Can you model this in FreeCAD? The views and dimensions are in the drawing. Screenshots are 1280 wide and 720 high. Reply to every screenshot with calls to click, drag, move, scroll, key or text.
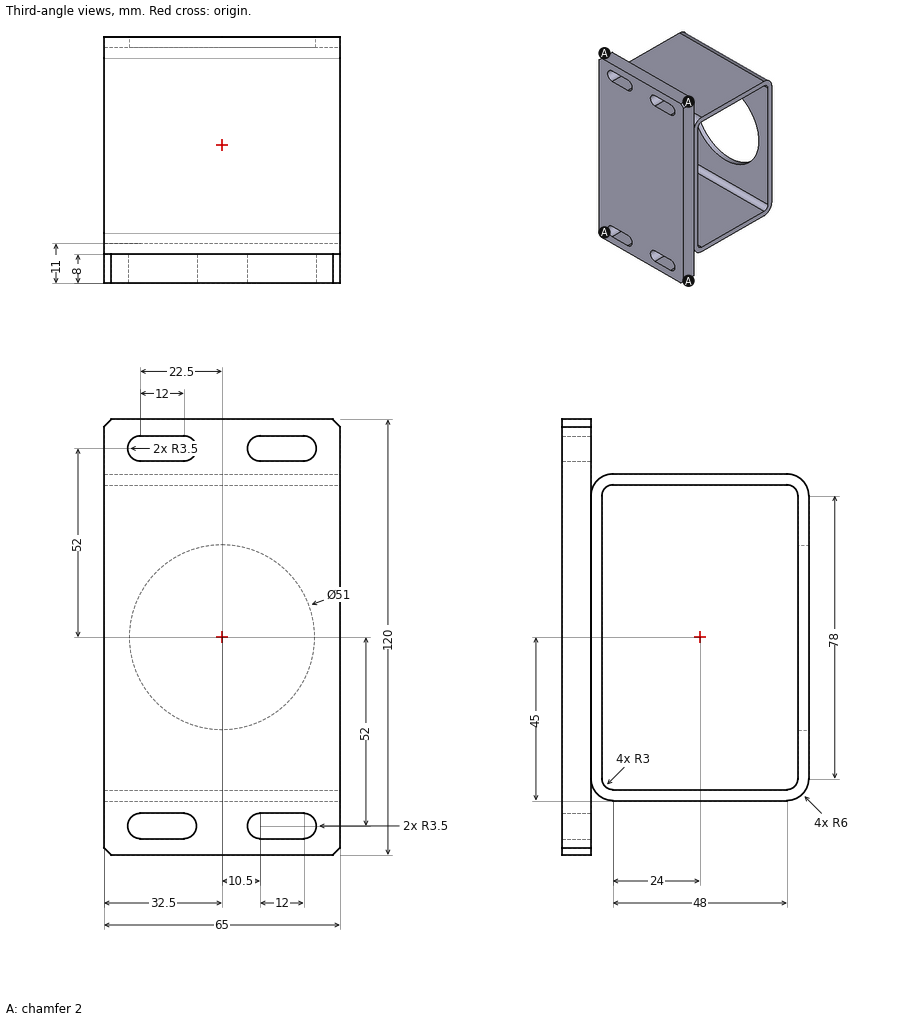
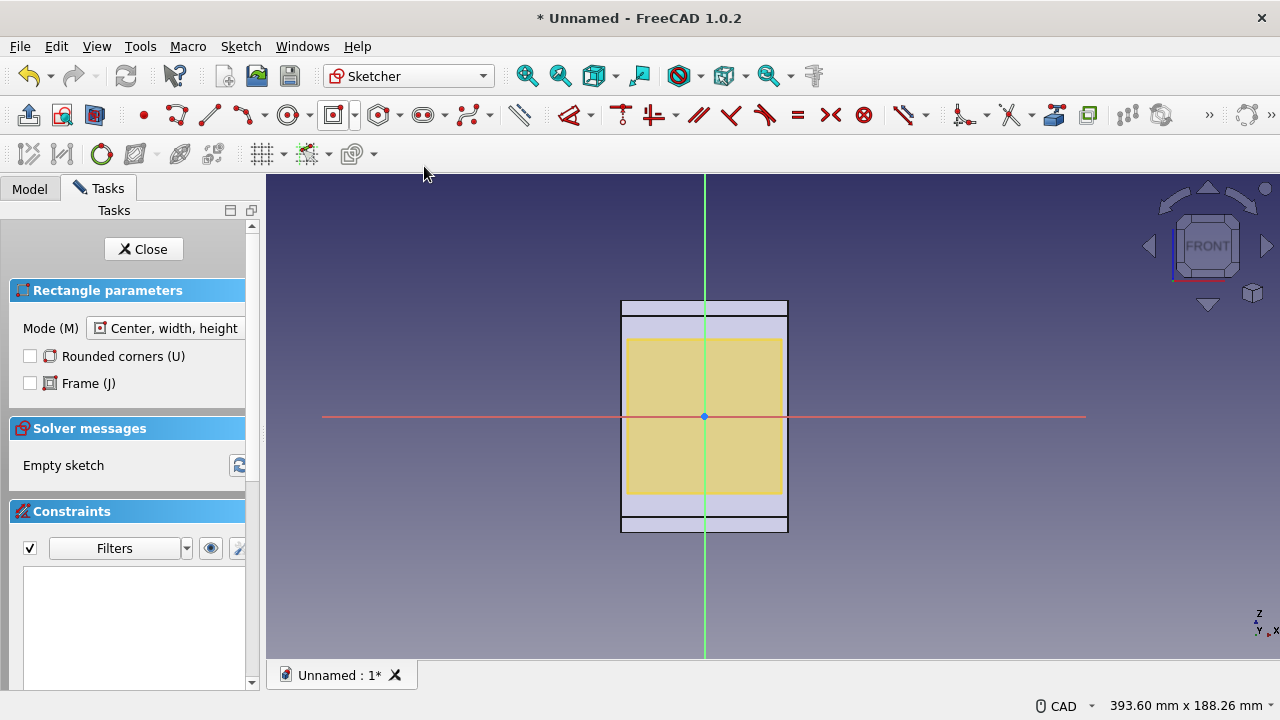
click(705, 417)
move(788, 262)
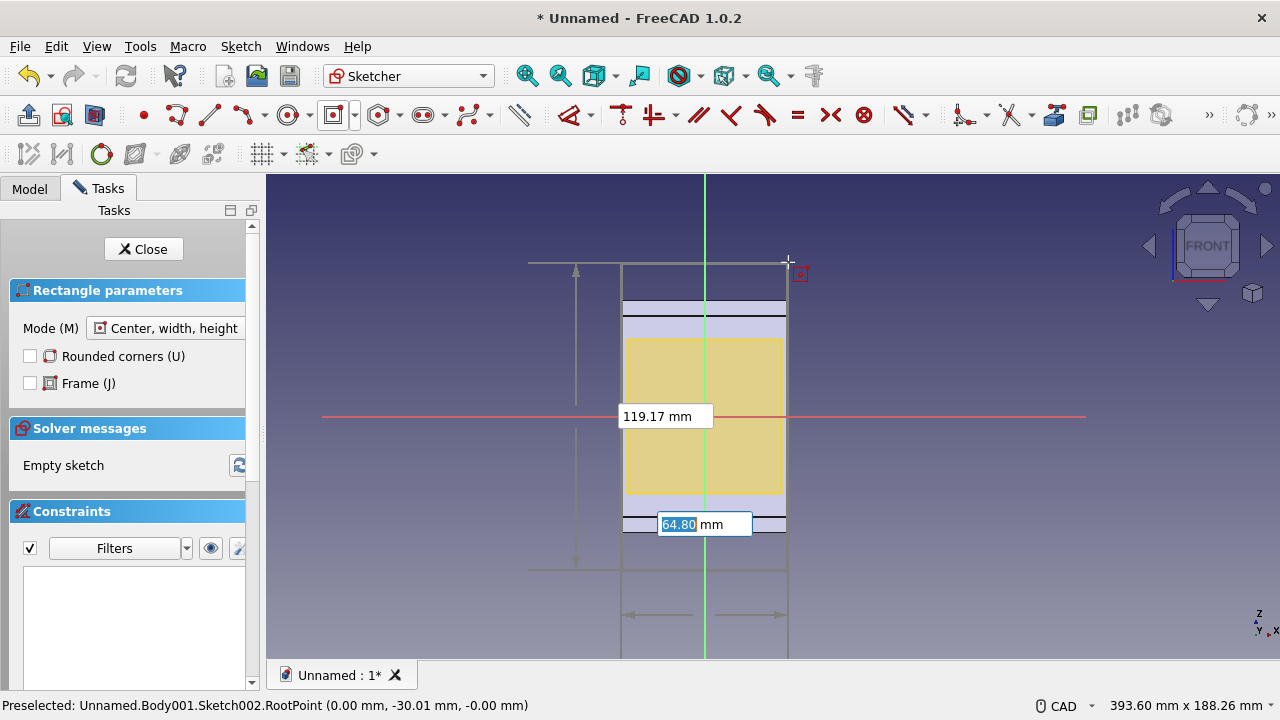
text(65)
key(Tab)
text(120)
key(Return)
key(Escape)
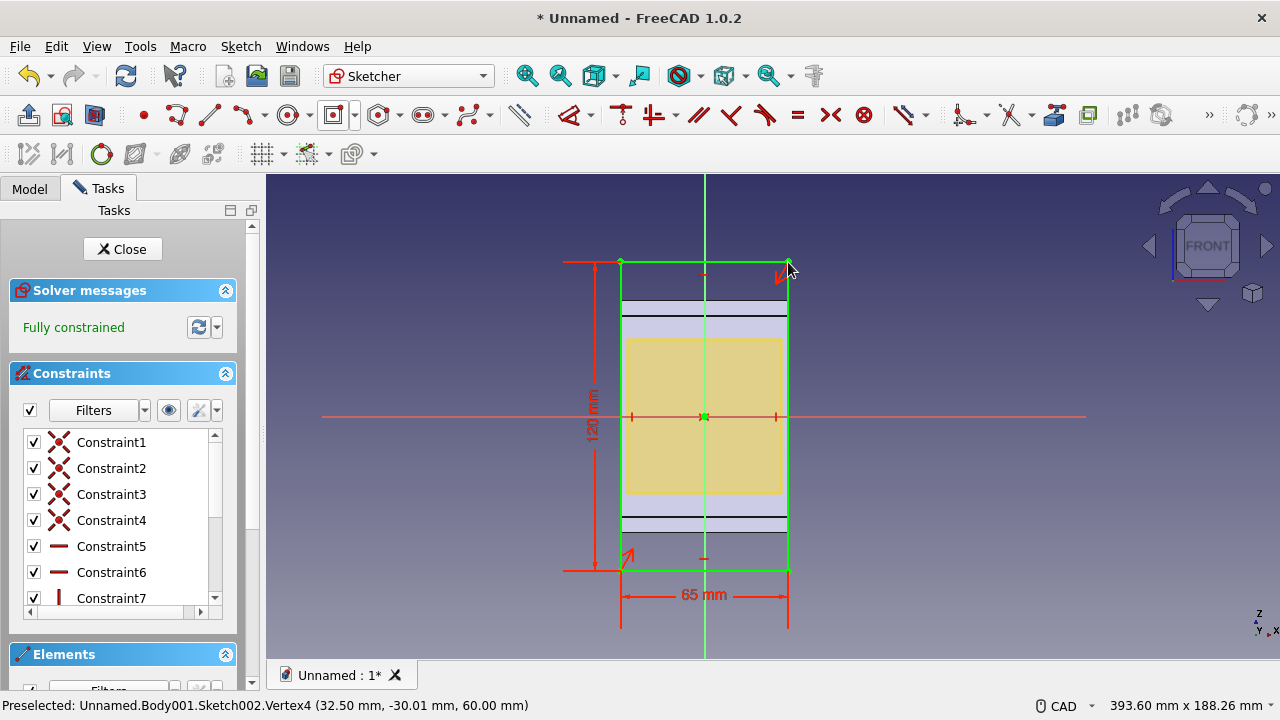
click(123, 249)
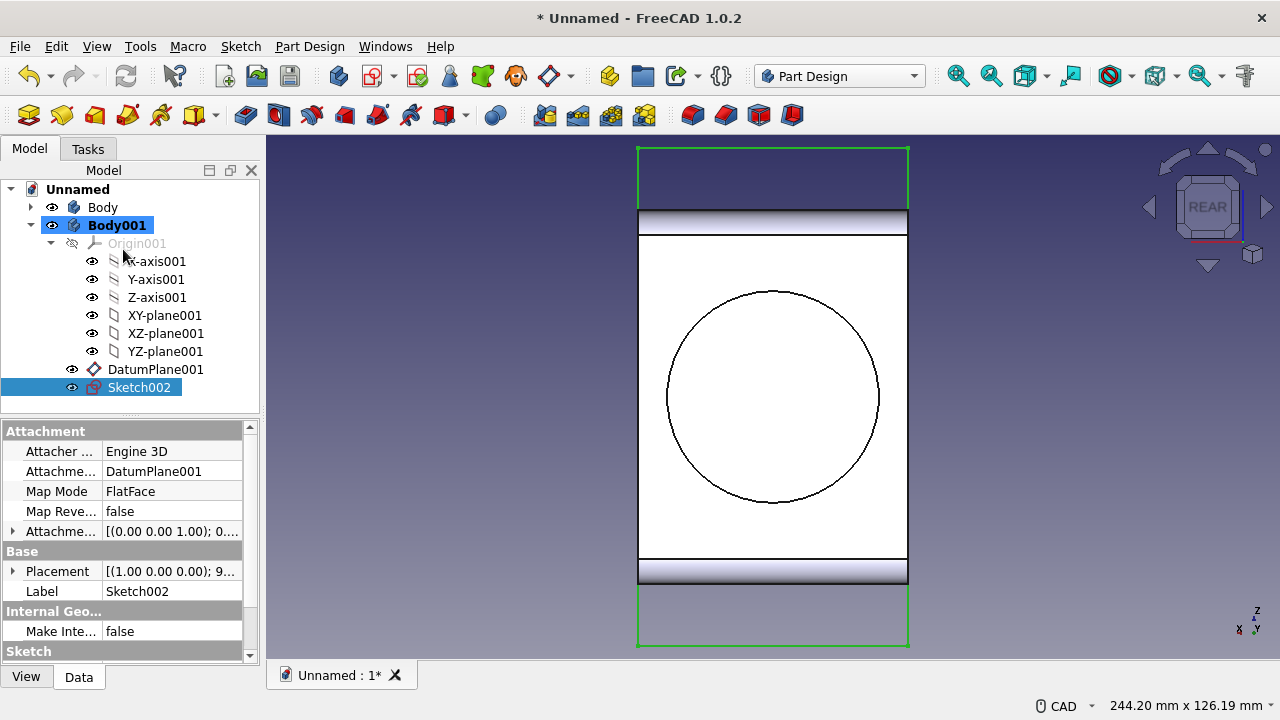
click(29, 116)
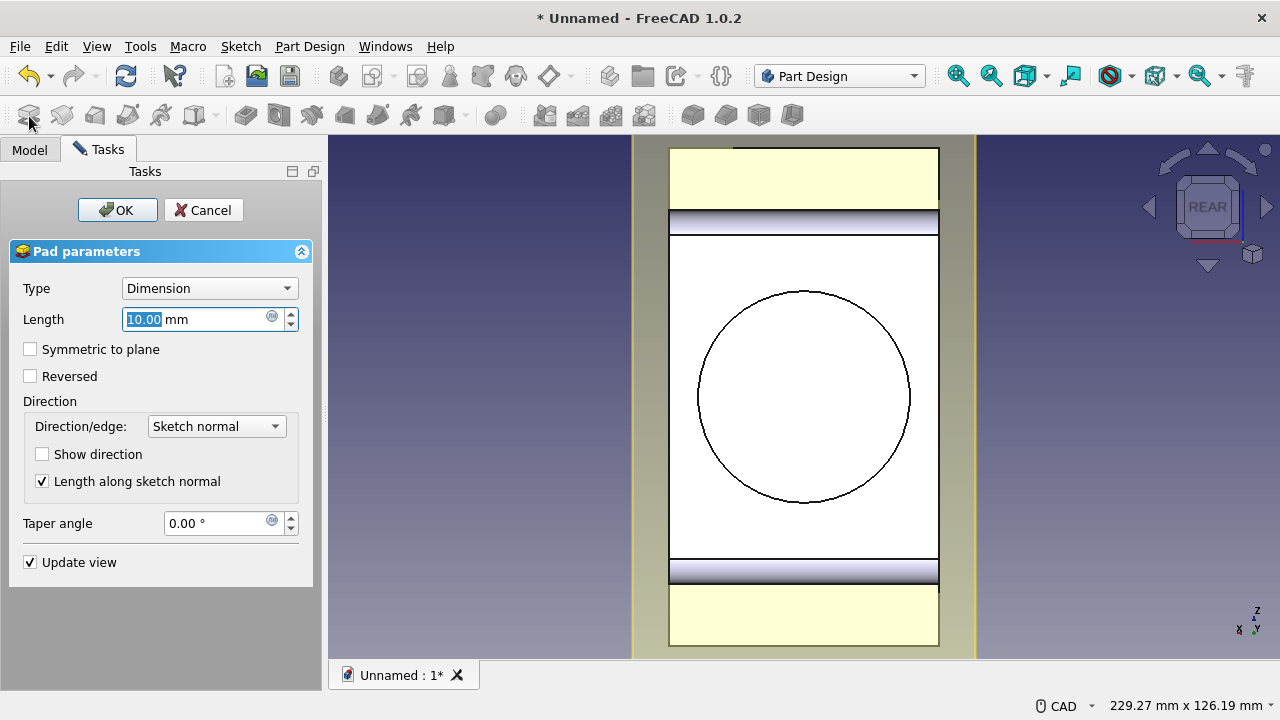
text(8)
key(Tab)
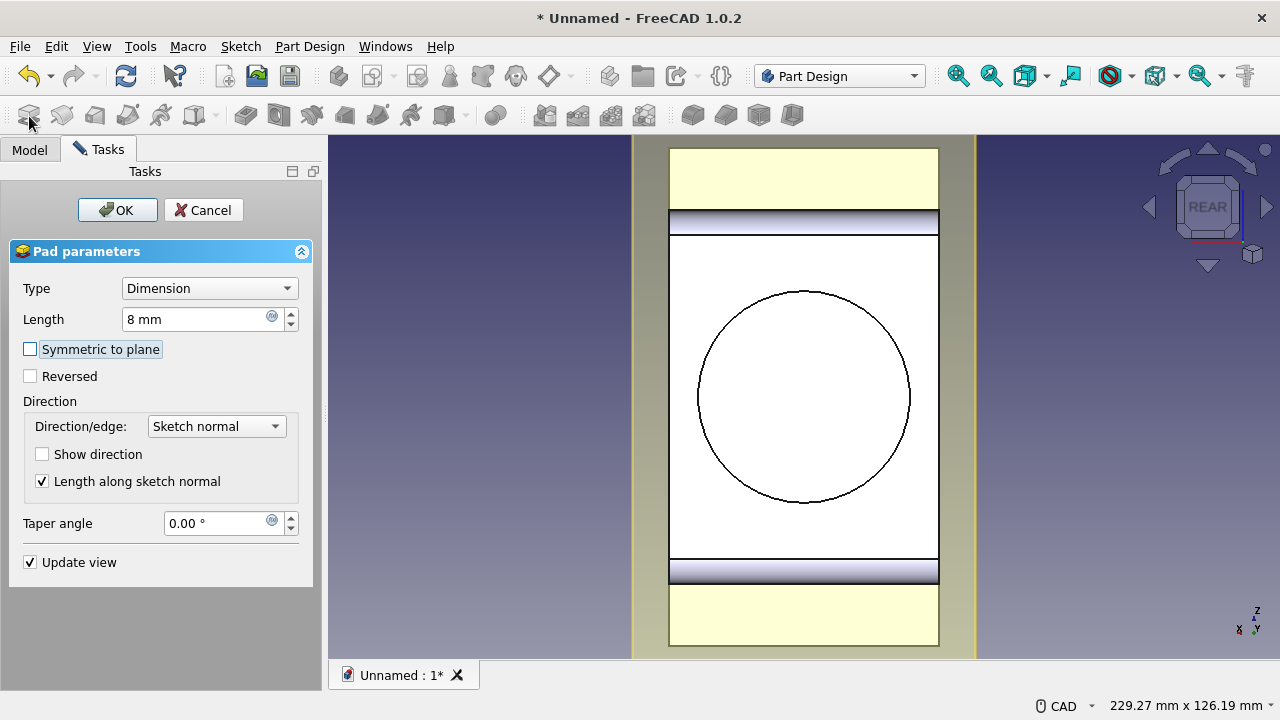
click(118, 210)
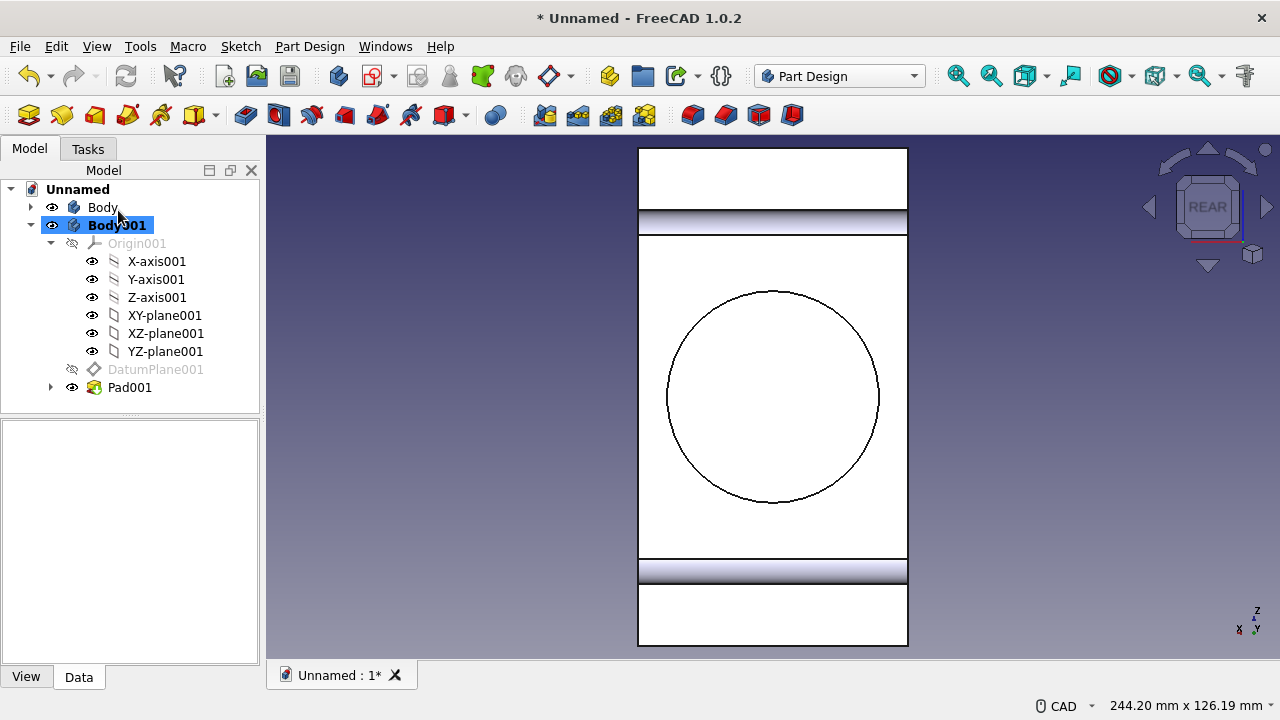
key(0)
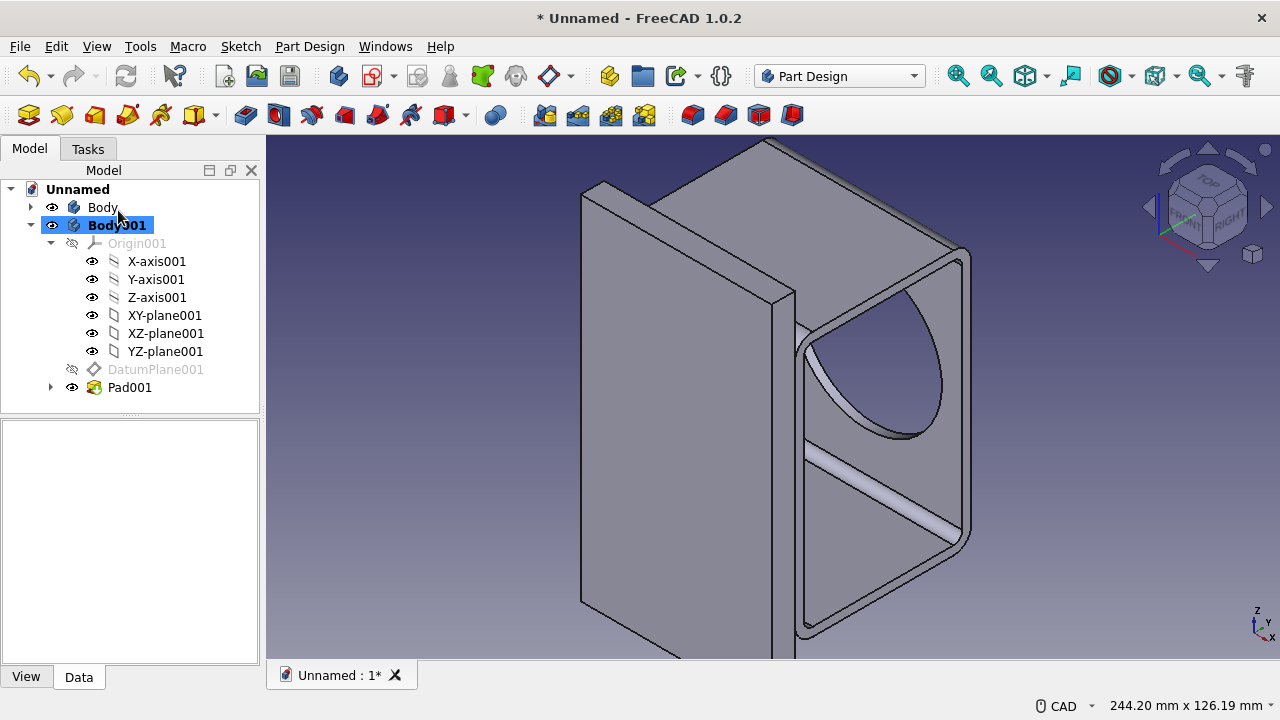
click(959, 76)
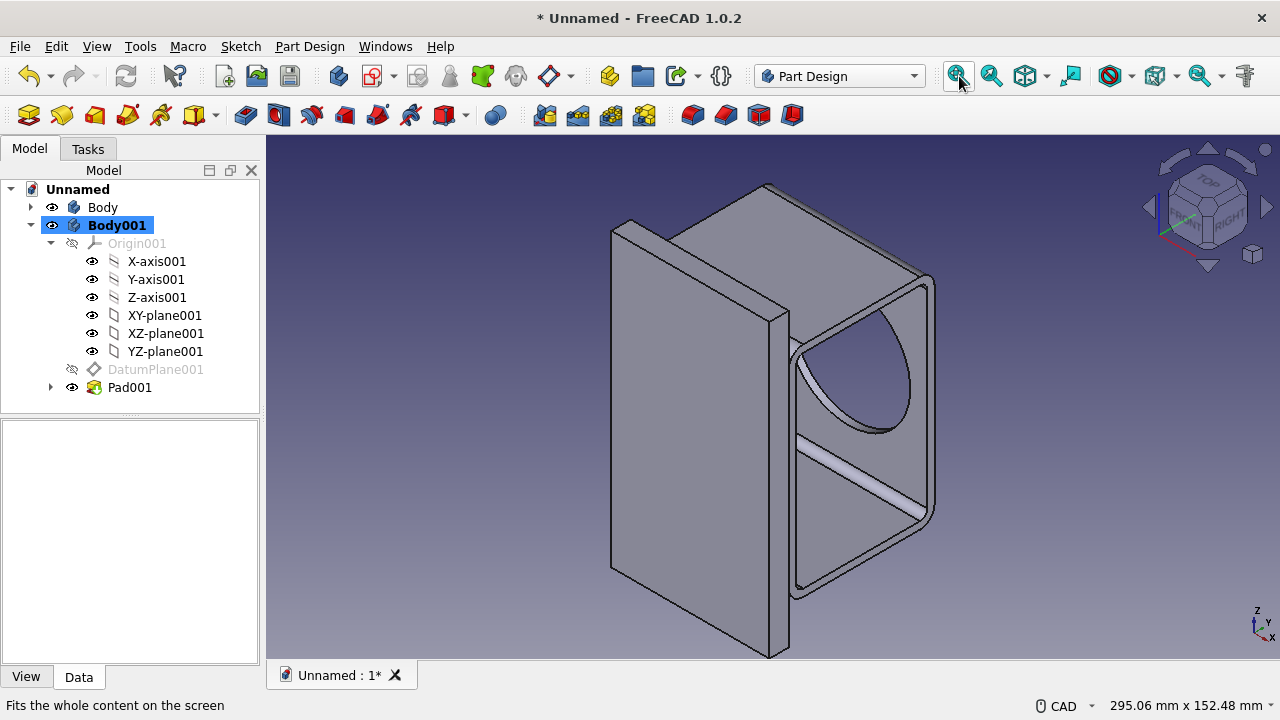
click(690, 396)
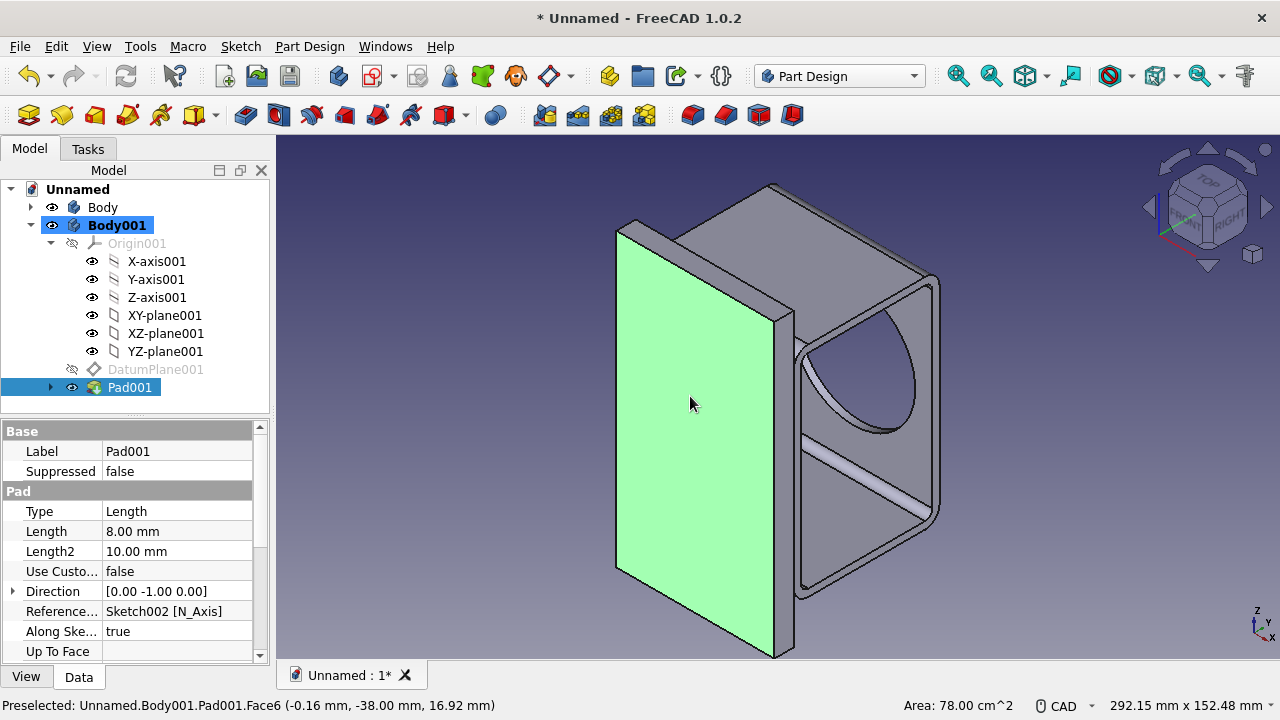
click(372, 76)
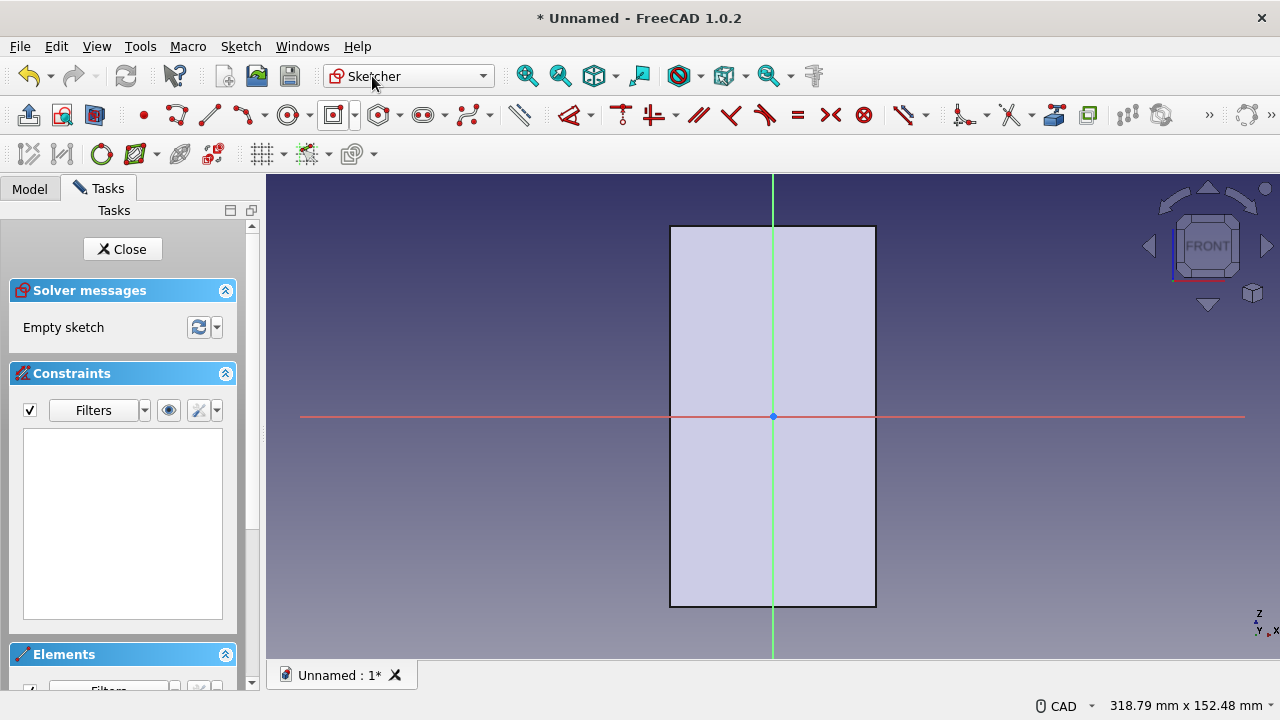
scroll(723, 230, up, 11)